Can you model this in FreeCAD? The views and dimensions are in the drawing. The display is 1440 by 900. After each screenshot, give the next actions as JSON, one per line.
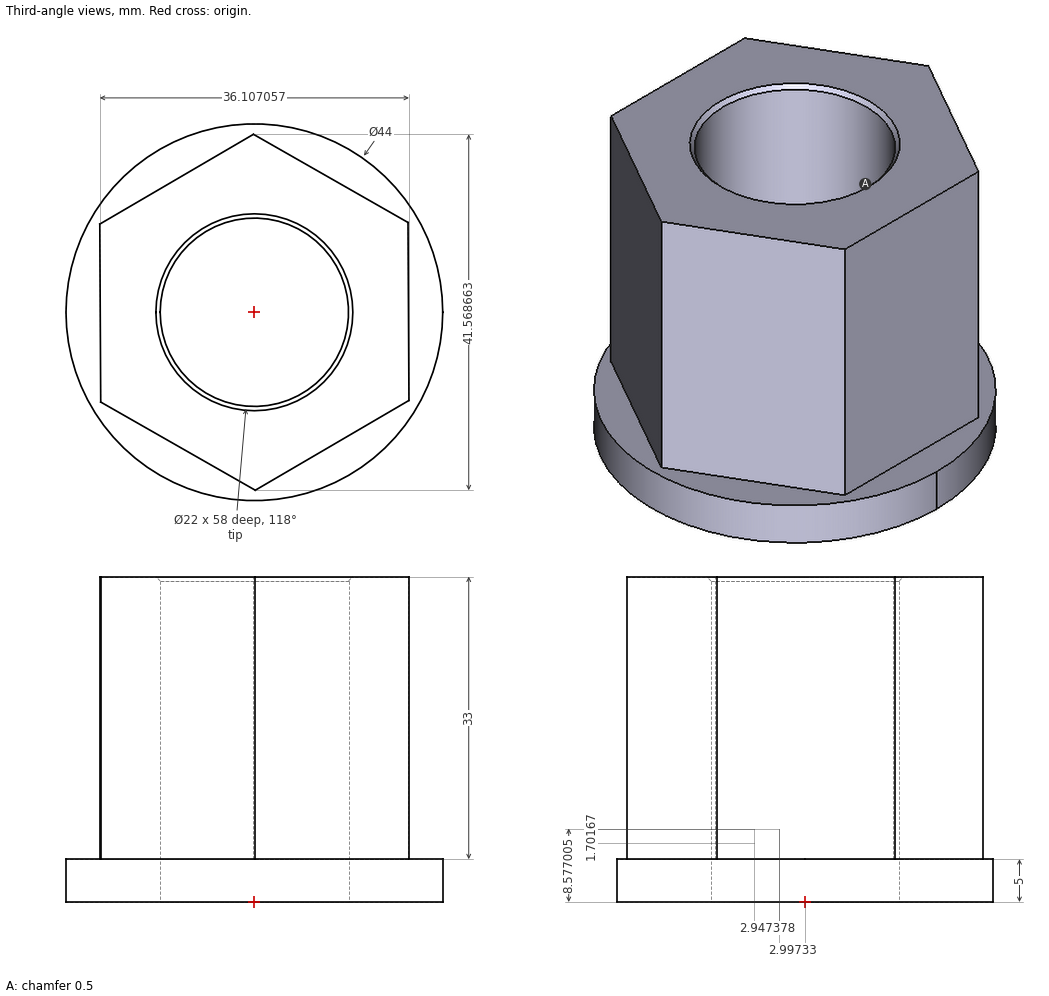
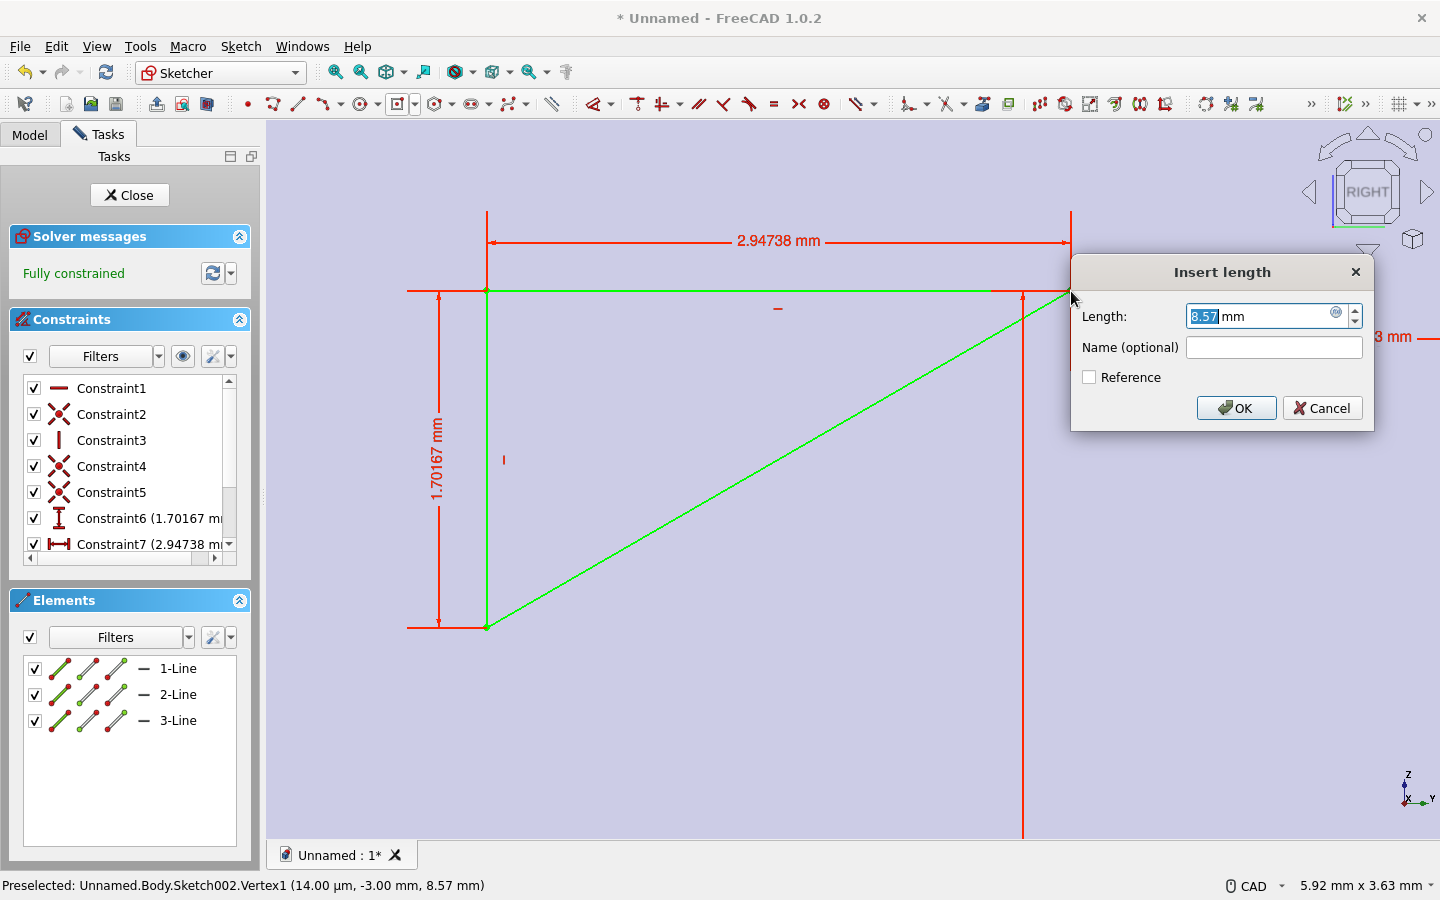
{"action": "type", "text": "8.577005"}
{"action": "key", "text": "Return"}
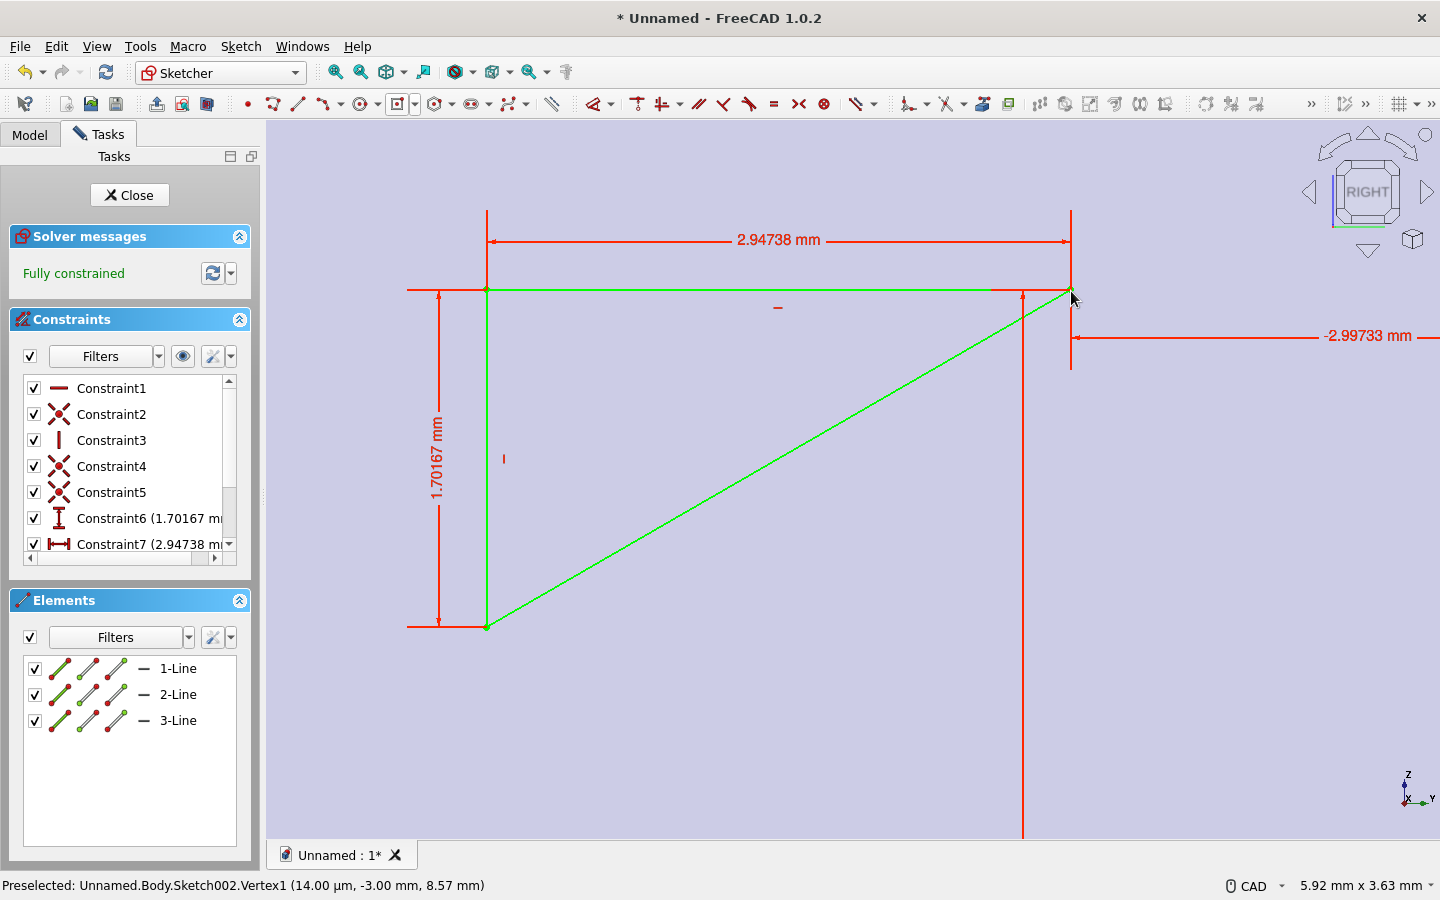
{"action": "left_click", "coordinate": [130, 195]}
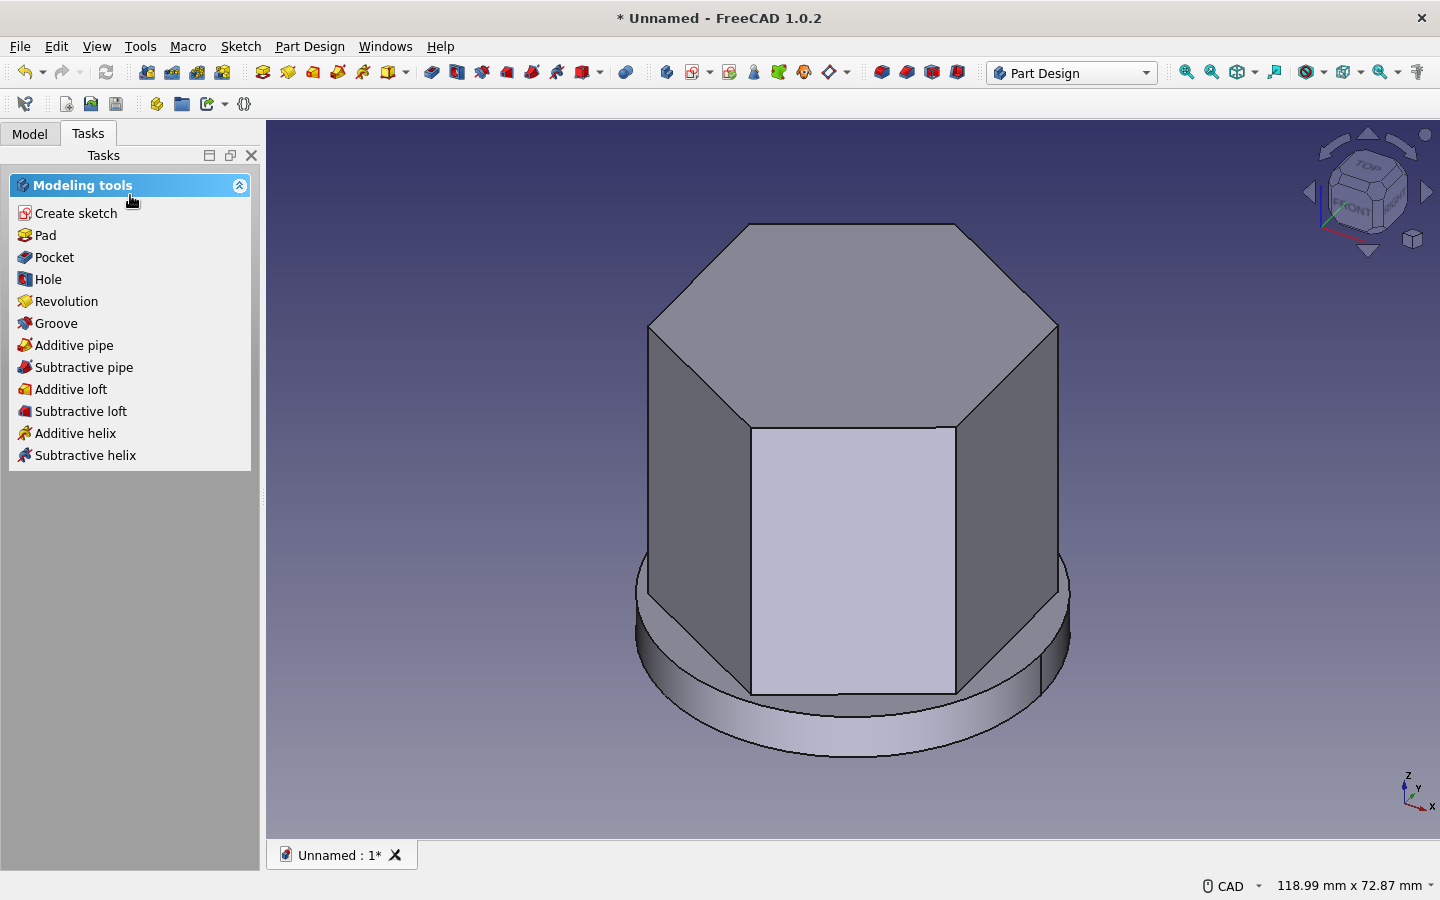
{"action": "left_click", "coordinate": [482, 72]}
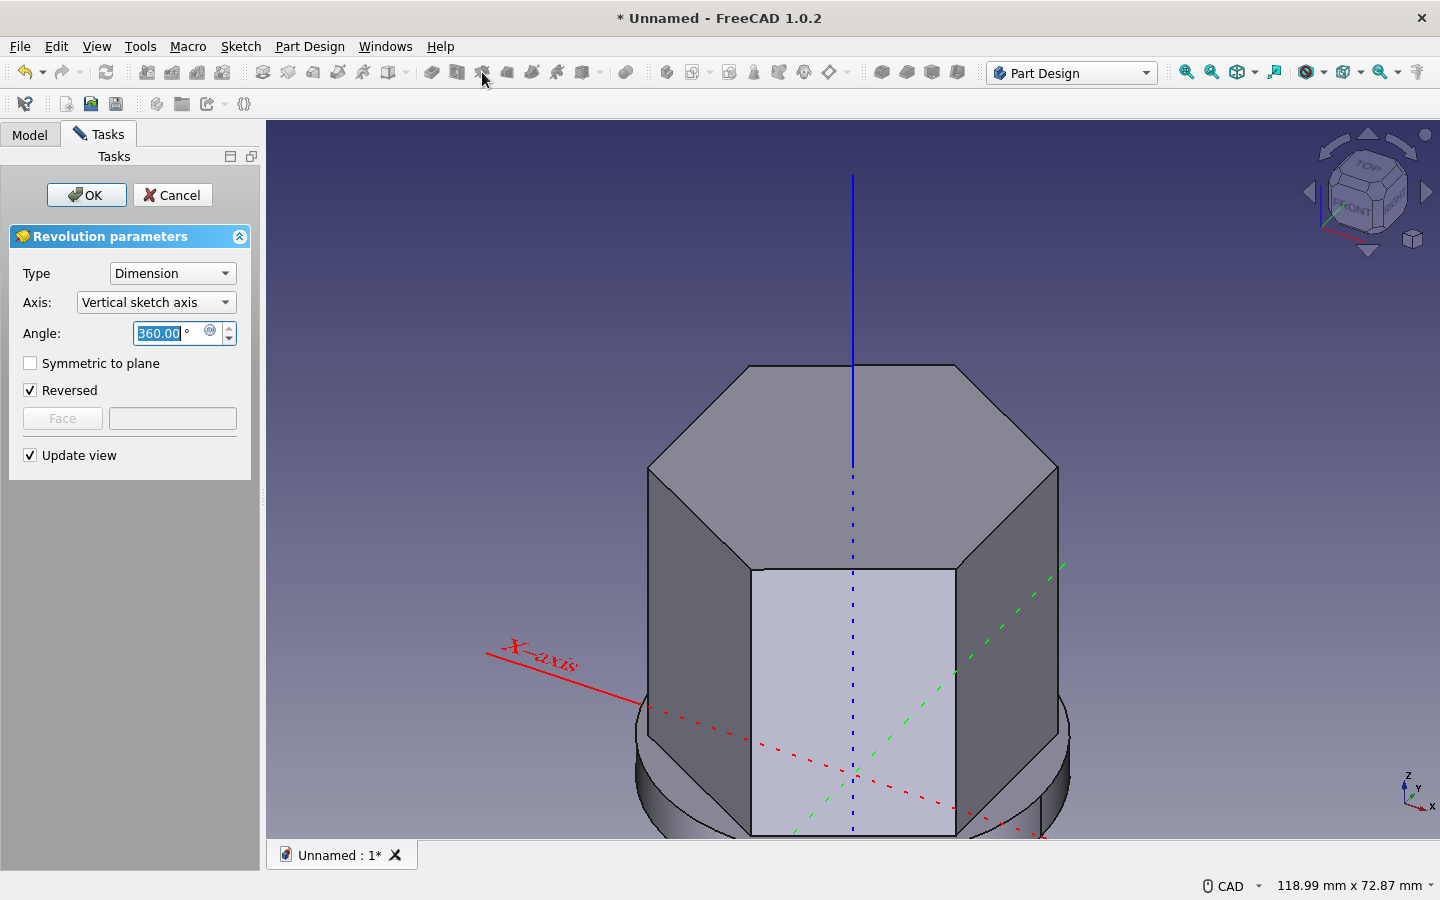
{"action": "left_click", "coordinate": [87, 195]}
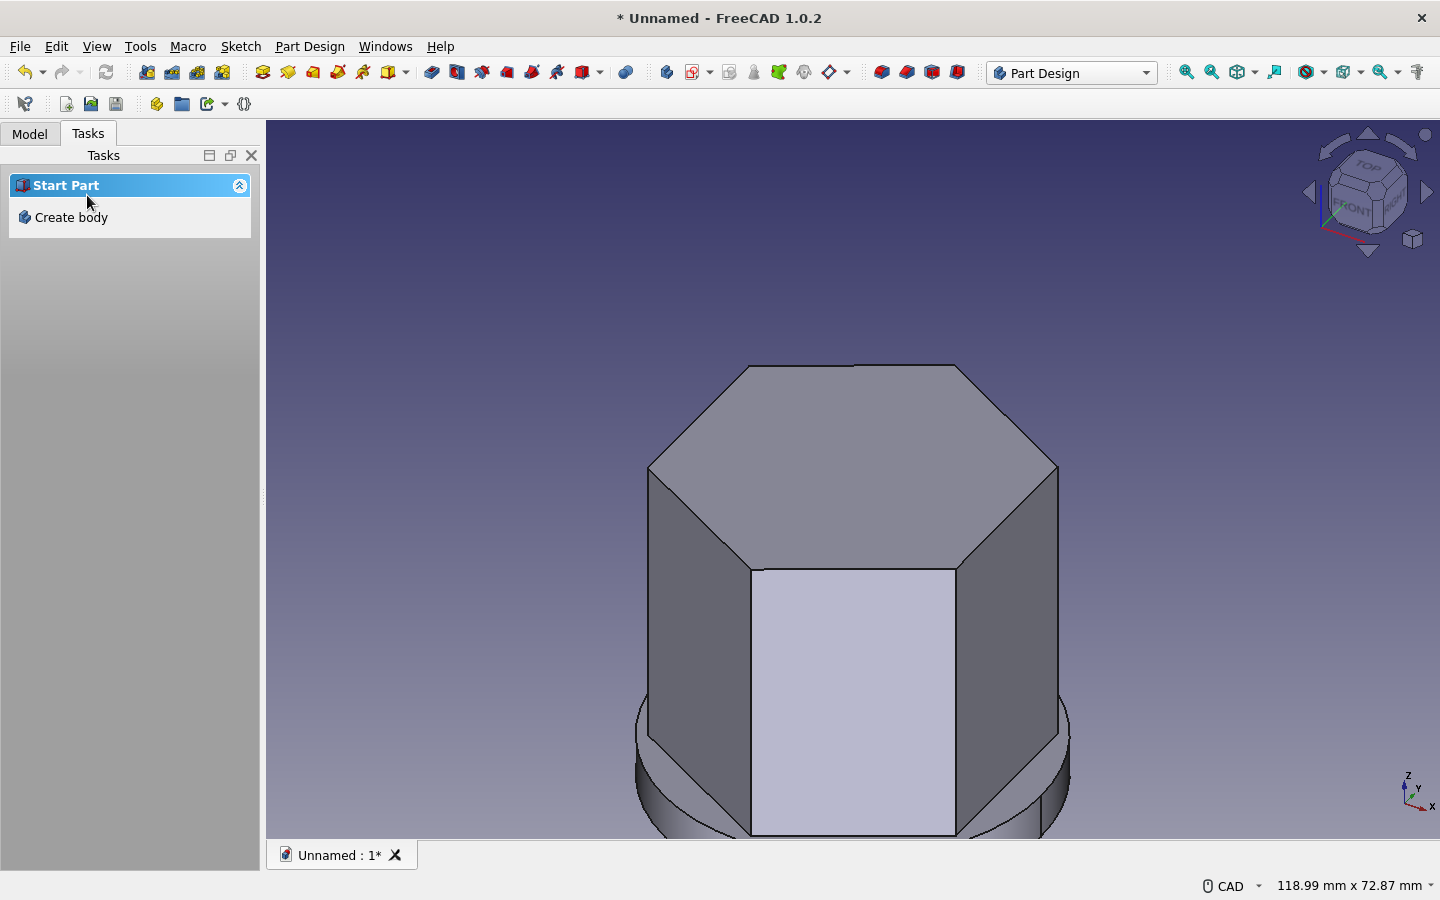
{"action": "key", "text": "v f"}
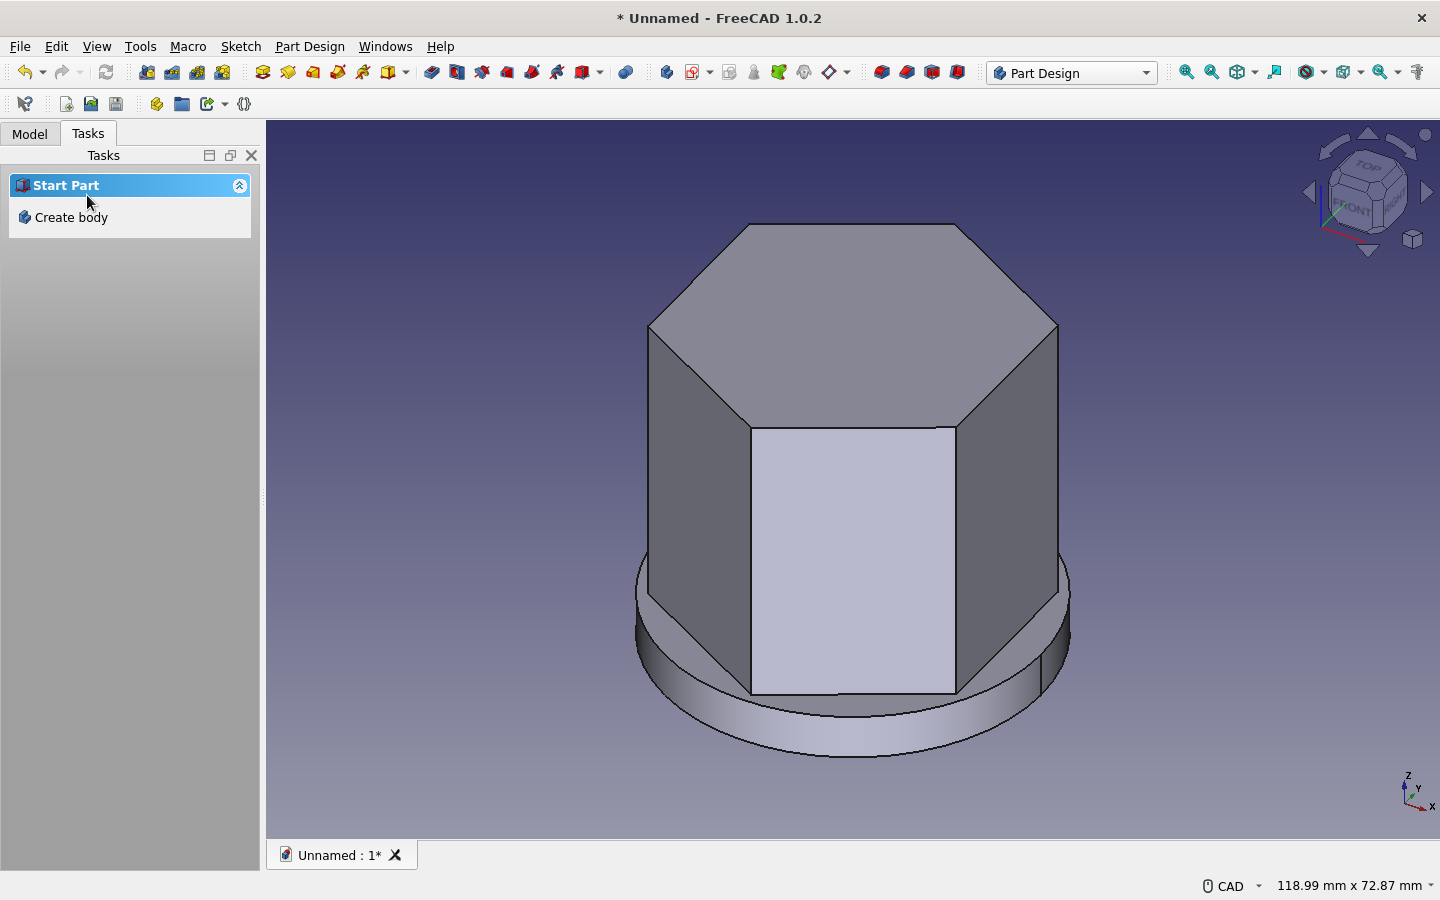
{"action": "left_click", "coordinate": [853, 325]}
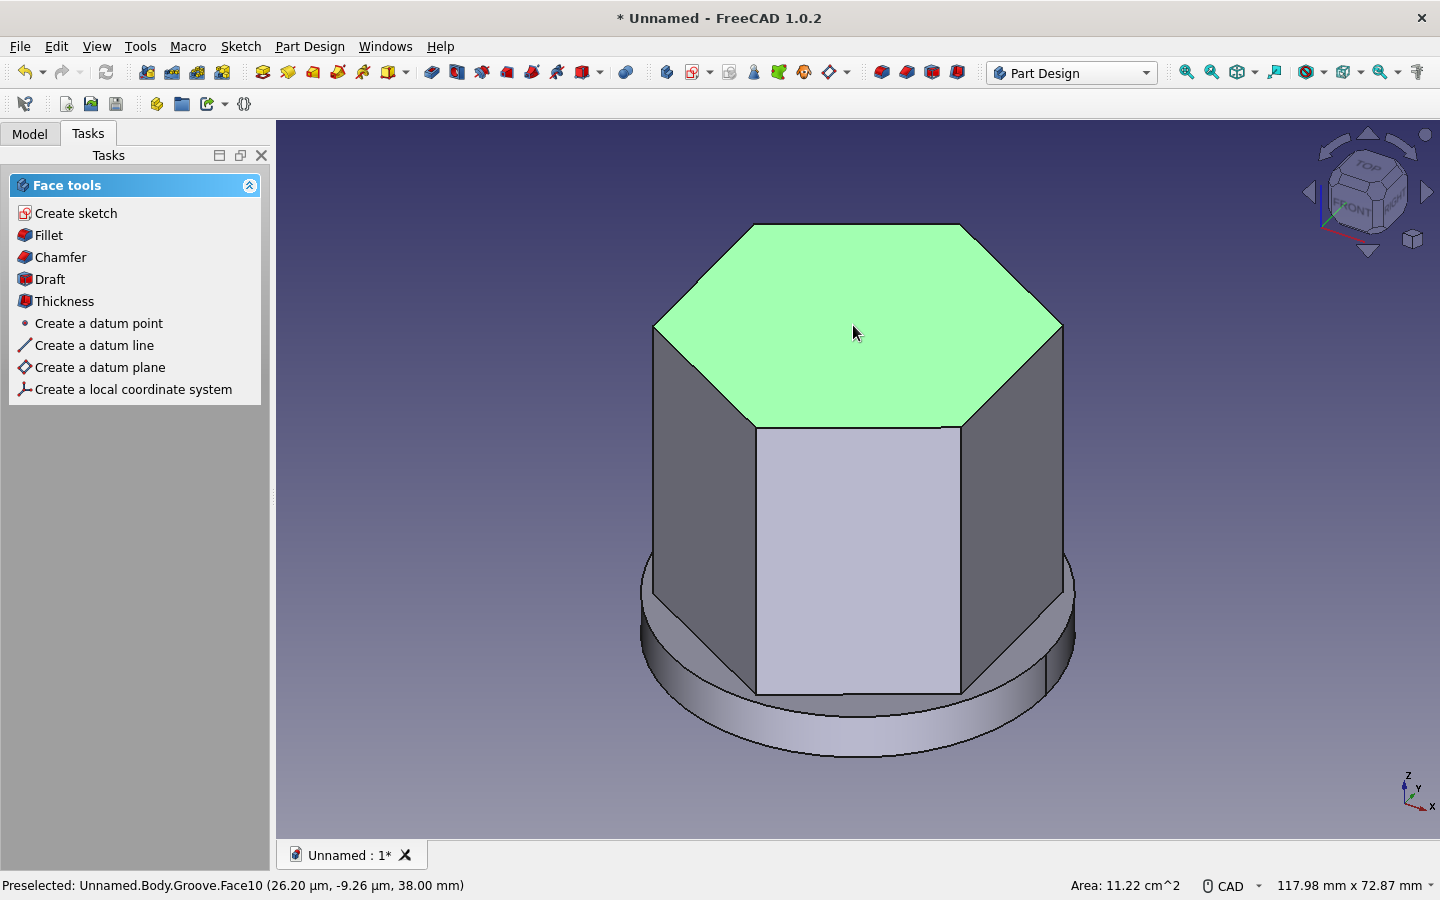
{"action": "left_click", "coordinate": [692, 72]}